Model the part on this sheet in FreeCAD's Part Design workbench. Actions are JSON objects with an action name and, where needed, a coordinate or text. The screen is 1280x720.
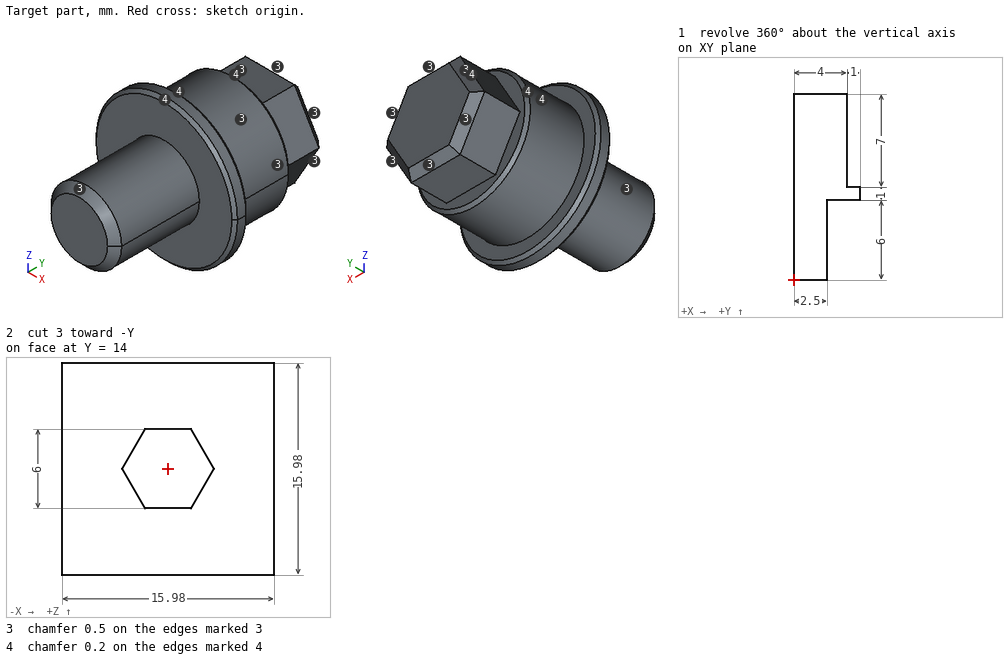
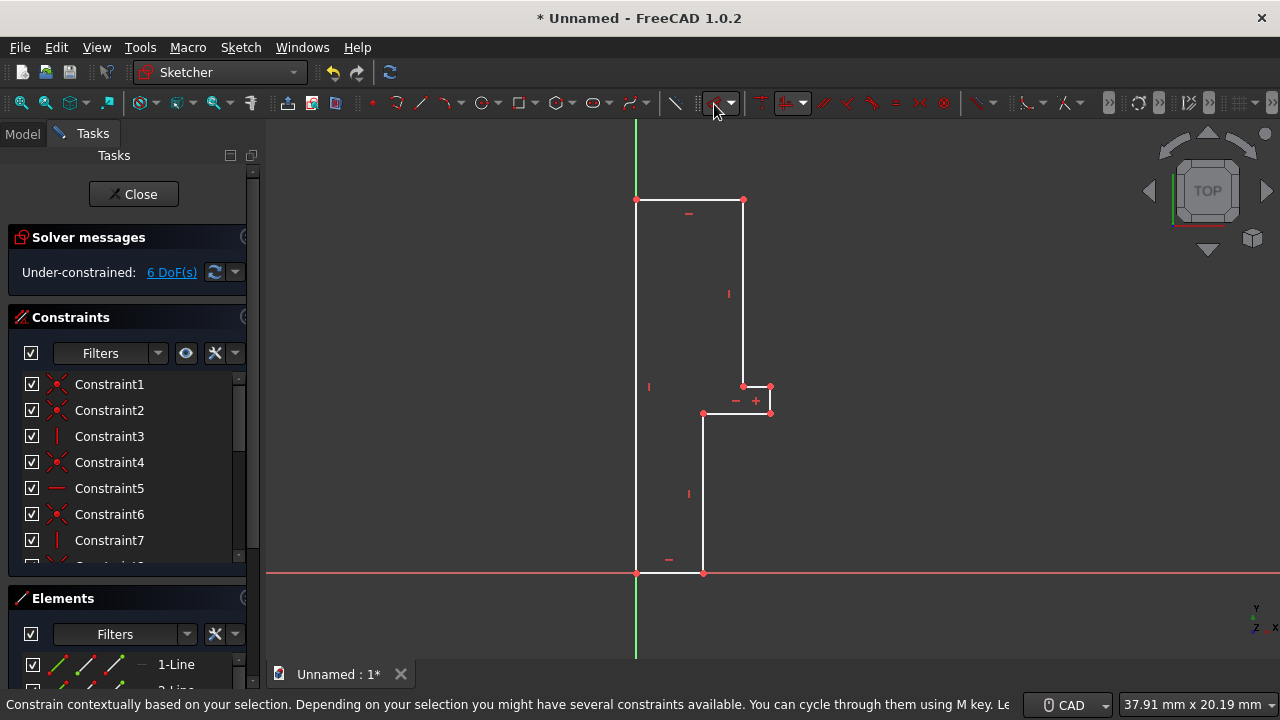
{"action": "left_click", "coordinate": [703, 525]}
{"action": "left_click", "coordinate": [669, 494]}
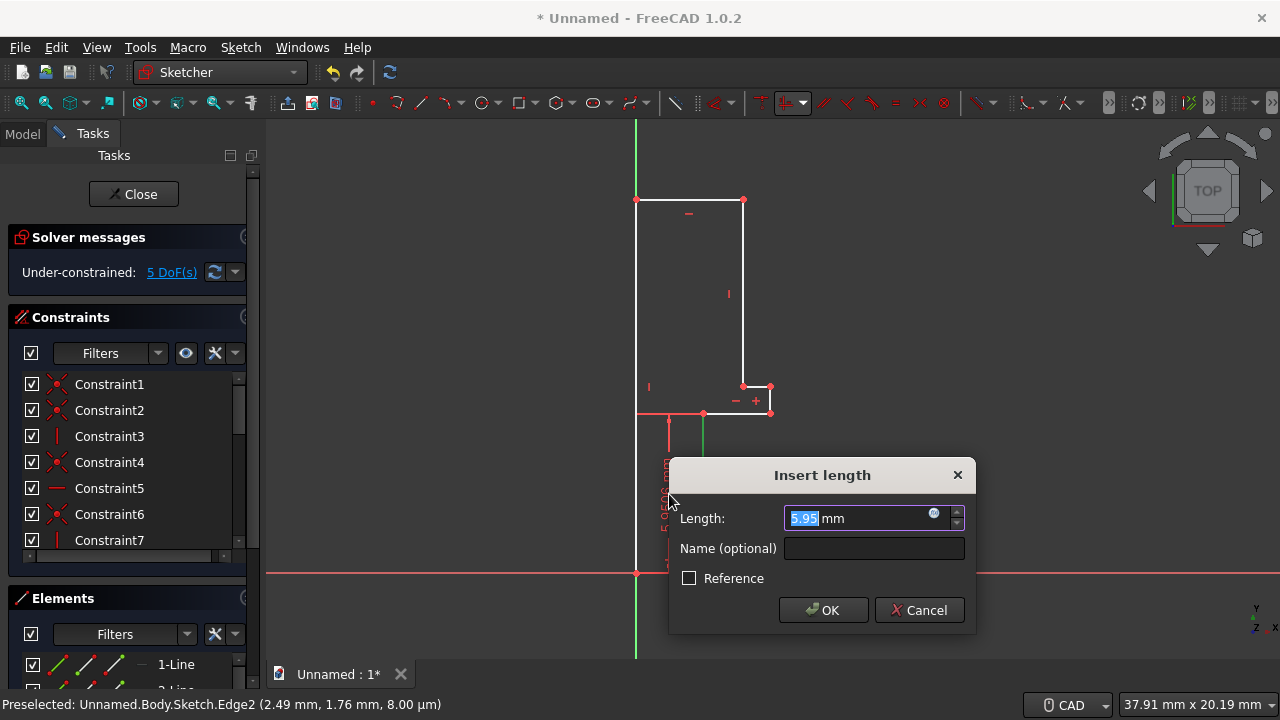
{"action": "type", "text": "6"}
{"action": "key", "text": "Return"}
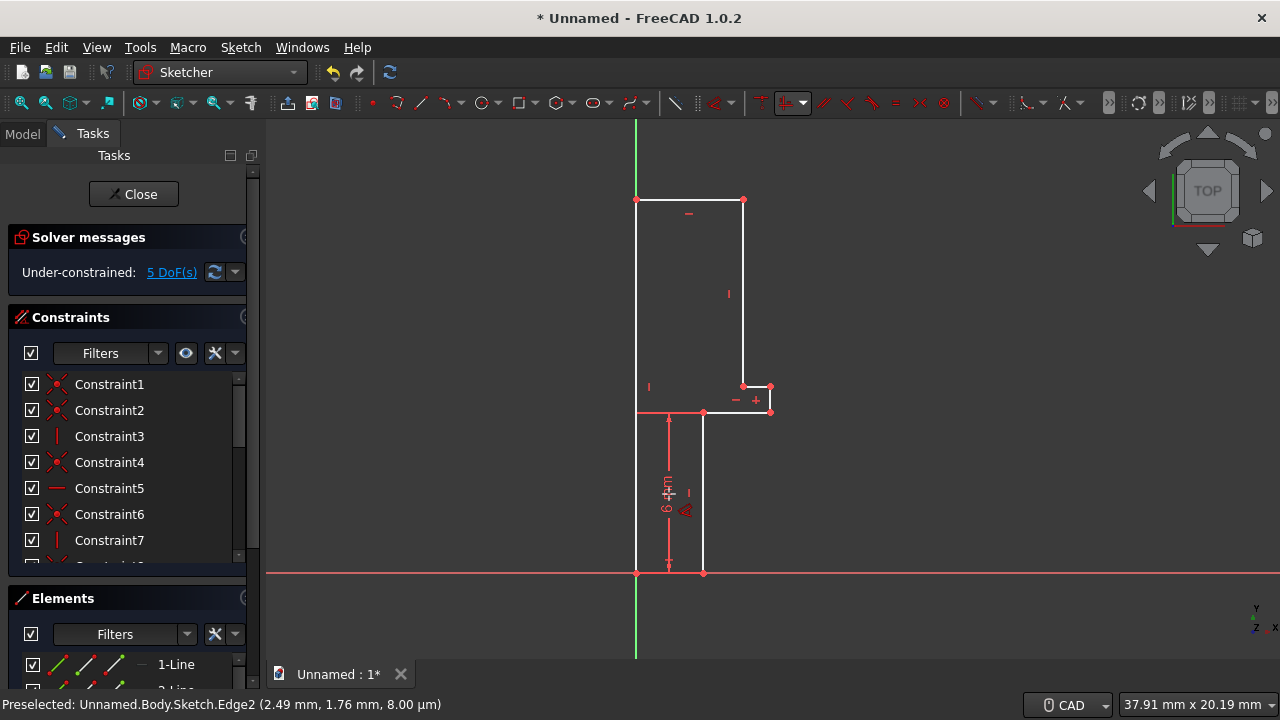
{"action": "scroll", "coordinate": [770, 402], "scroll_direction": "up", "scroll_amount": 2}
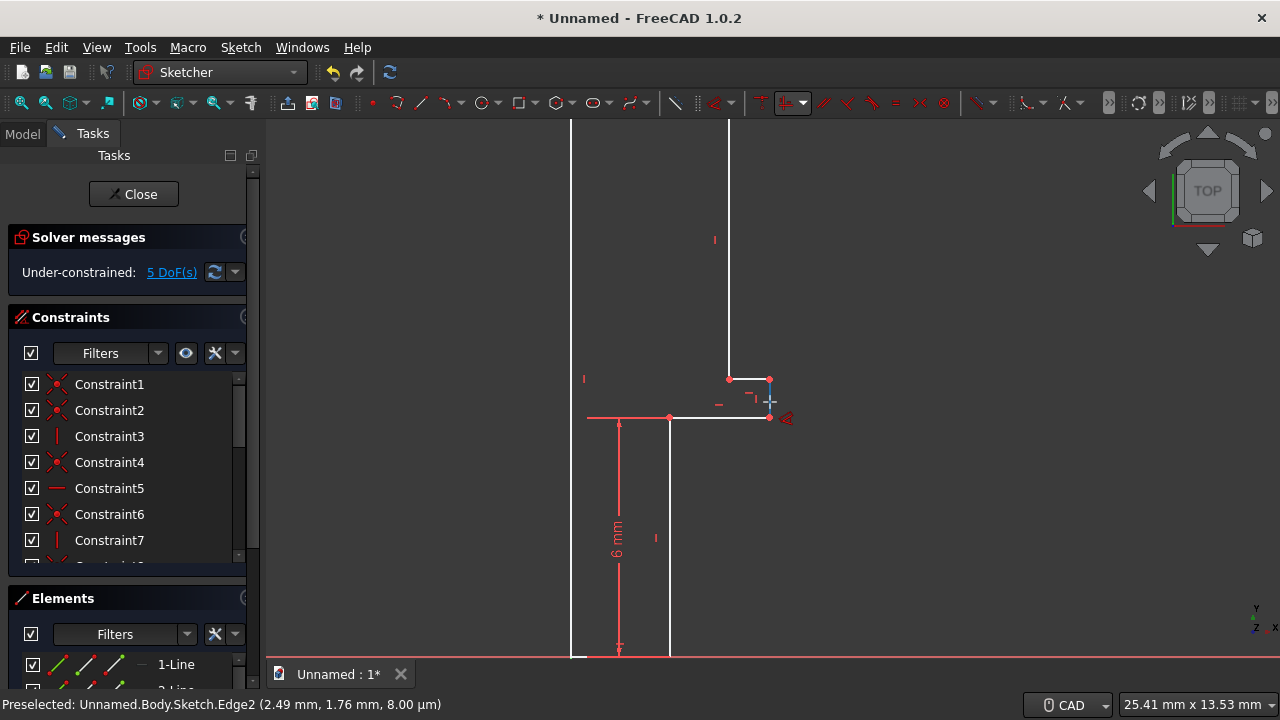
{"action": "left_click", "coordinate": [770, 402]}
{"action": "left_click", "coordinate": [804, 399]}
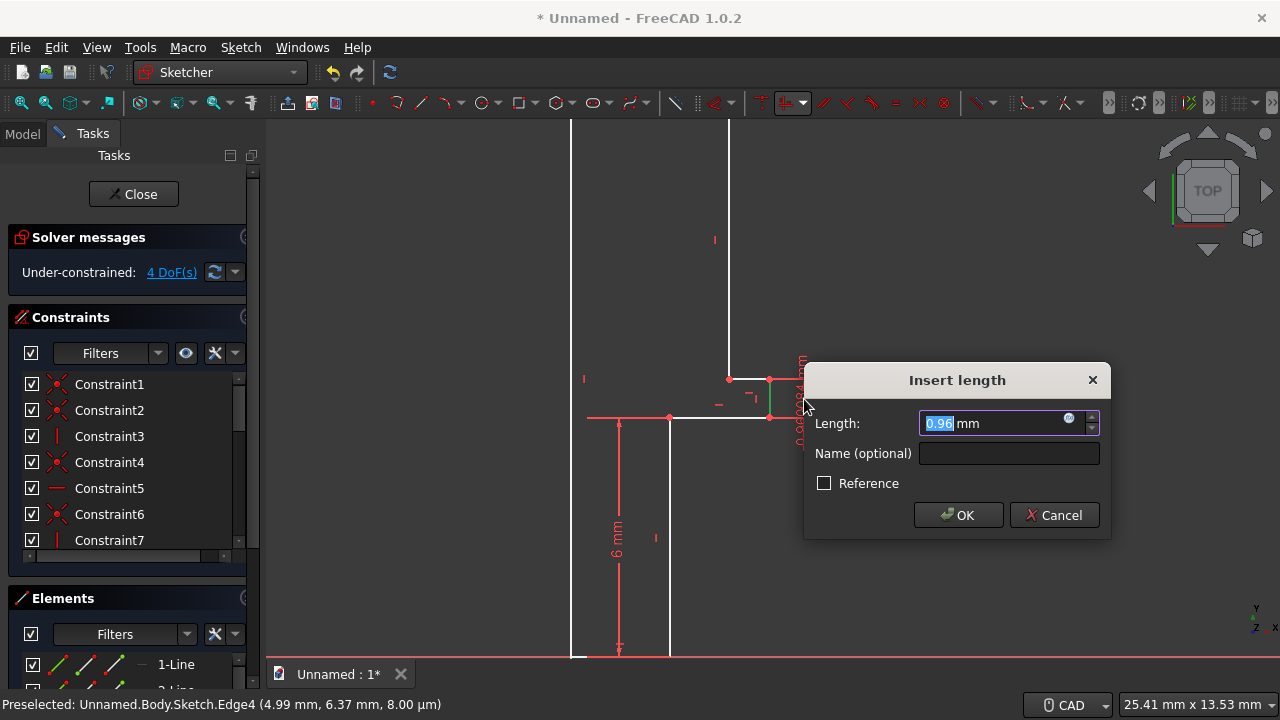
{"action": "type", "text": "1"}
{"action": "key", "text": "Return"}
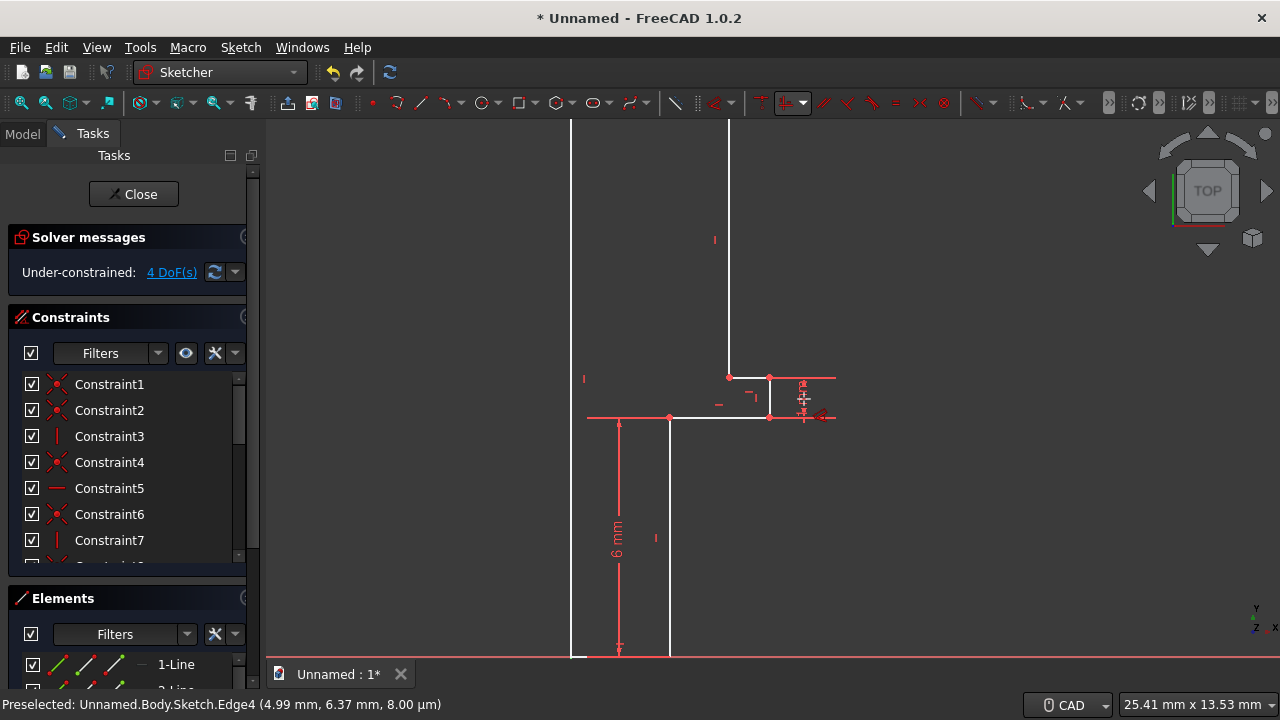
{"action": "left_click", "coordinate": [758, 378]}
{"action": "left_click", "coordinate": [750, 344]}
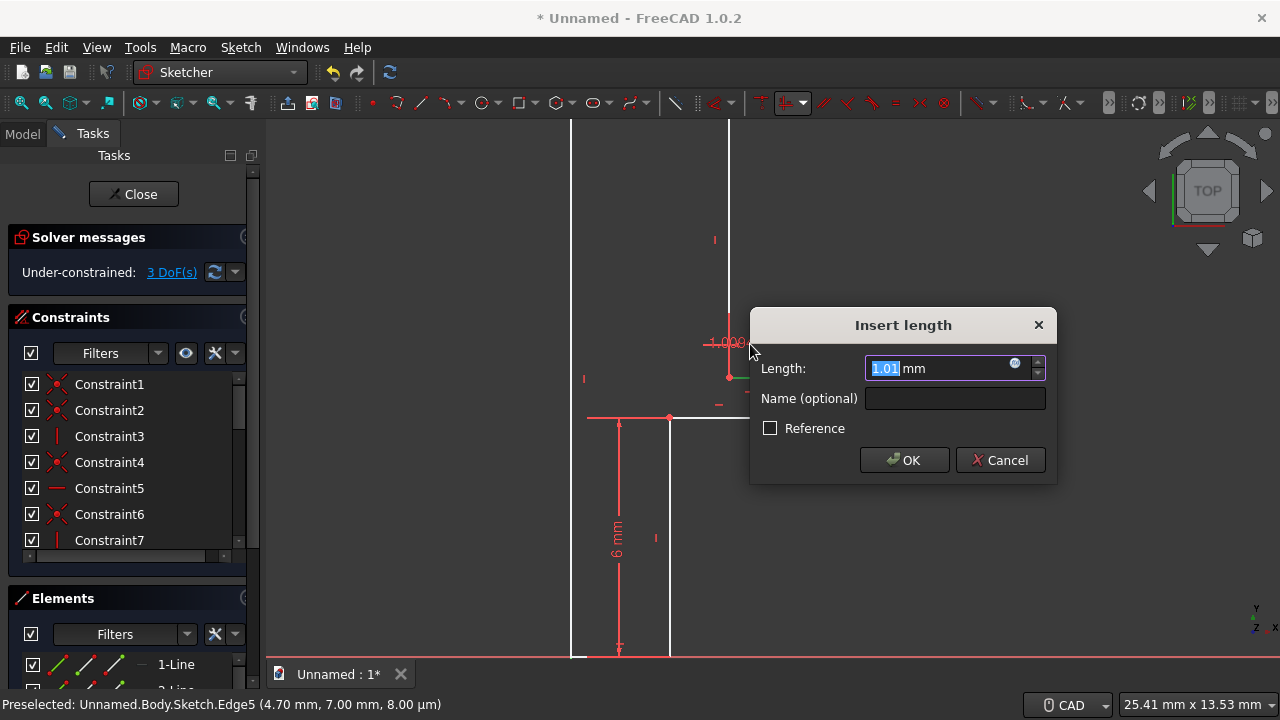
{"action": "type", "text": "1"}
{"action": "key", "text": "Return"}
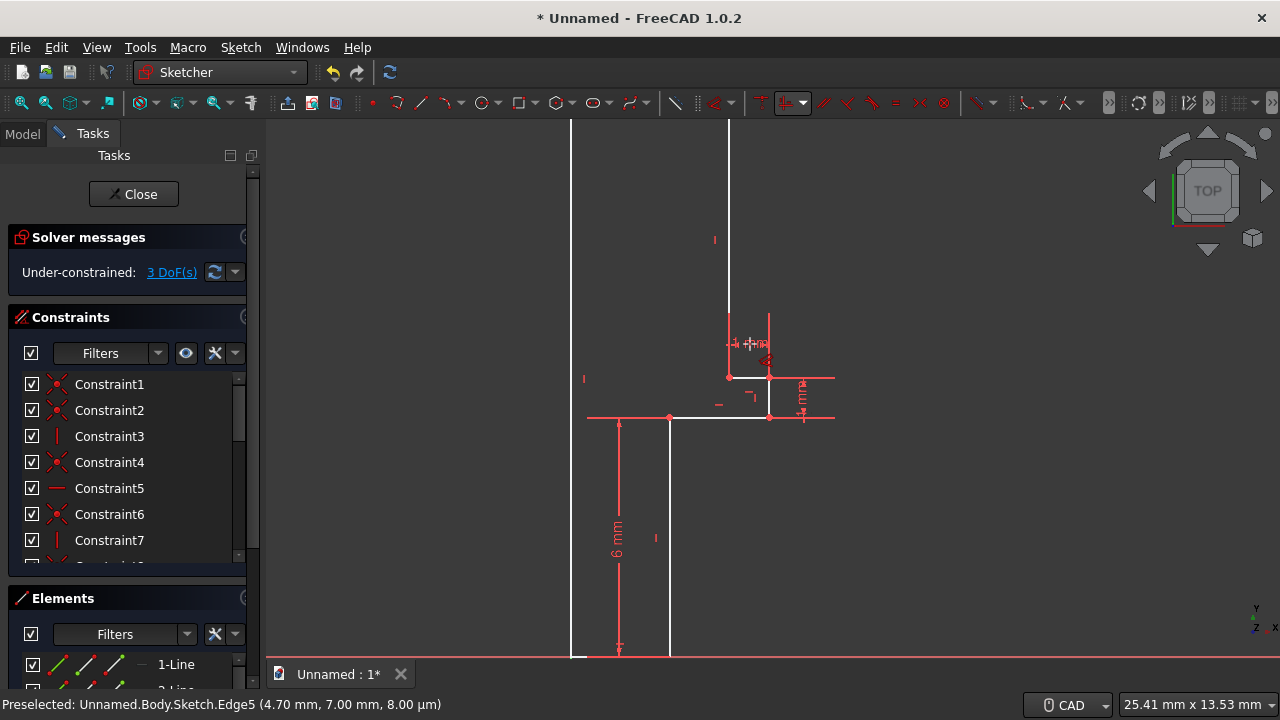
{"action": "left_click", "coordinate": [729, 295]}
{"action": "left_click", "coordinate": [763, 262]}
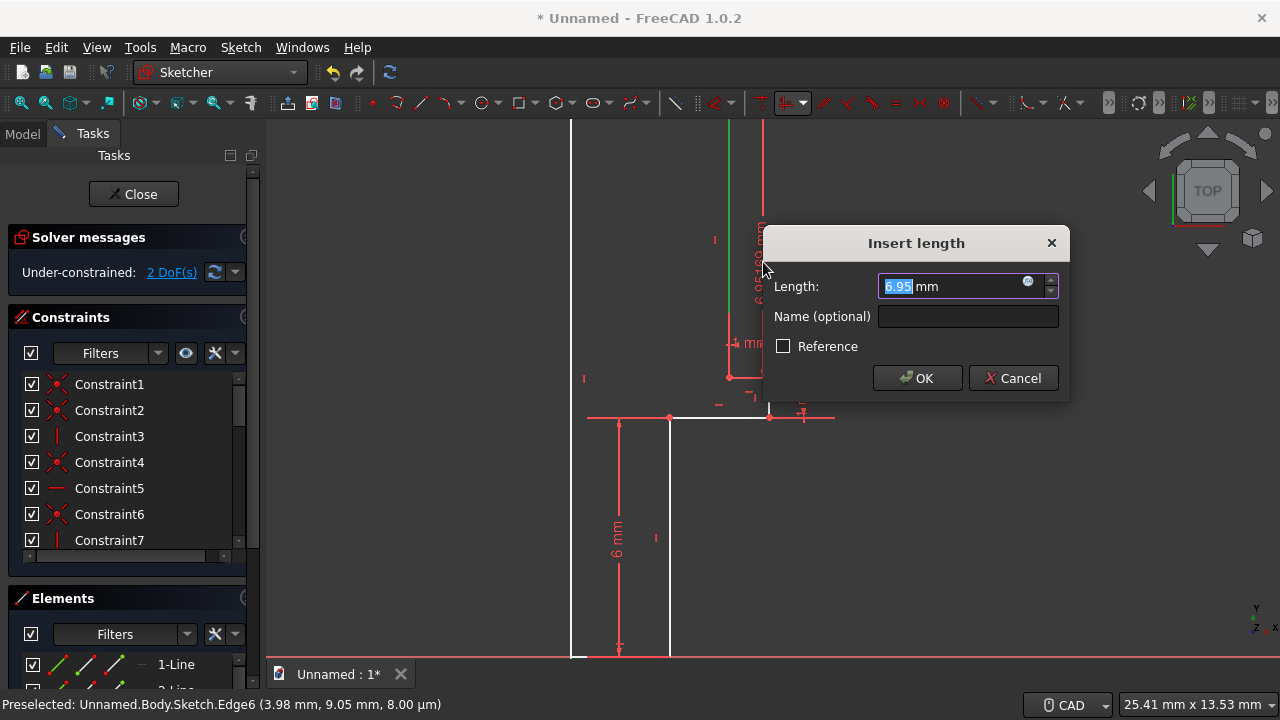
{"action": "type", "text": "7"}
{"action": "key", "text": "Return"}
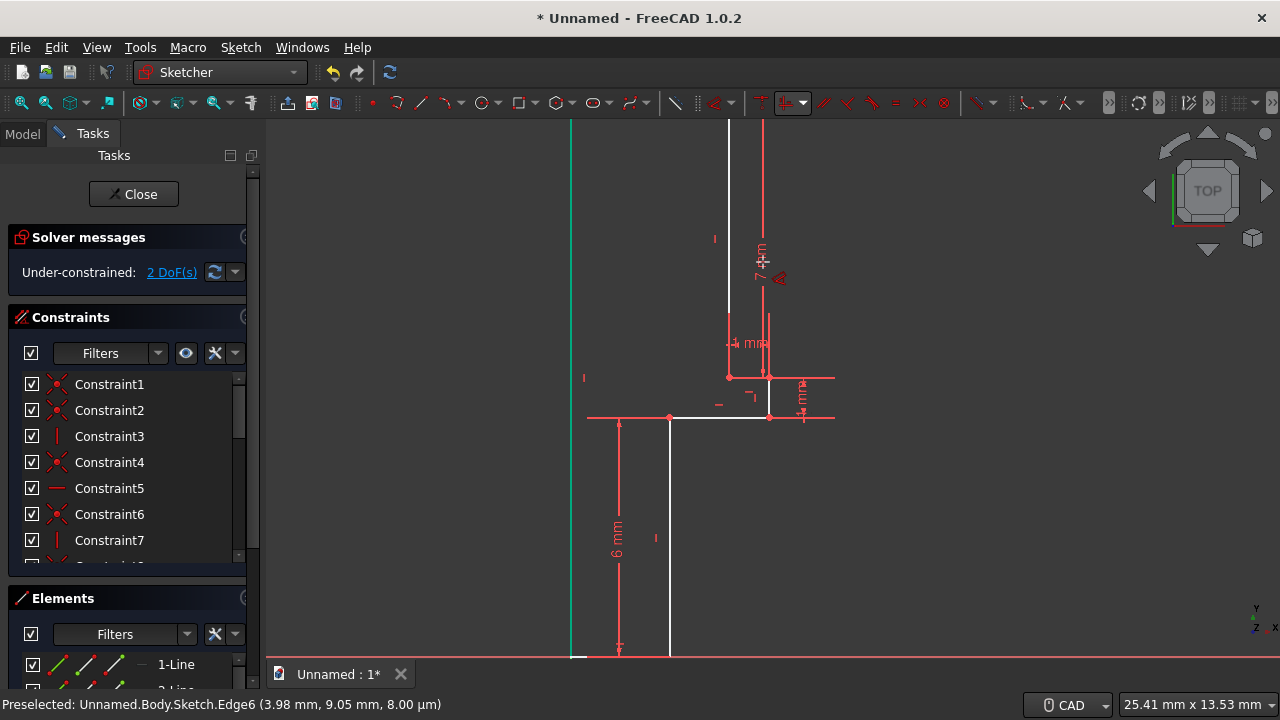
{"action": "scroll", "coordinate": [774, 412], "scroll_direction": "down", "scroll_amount": 2}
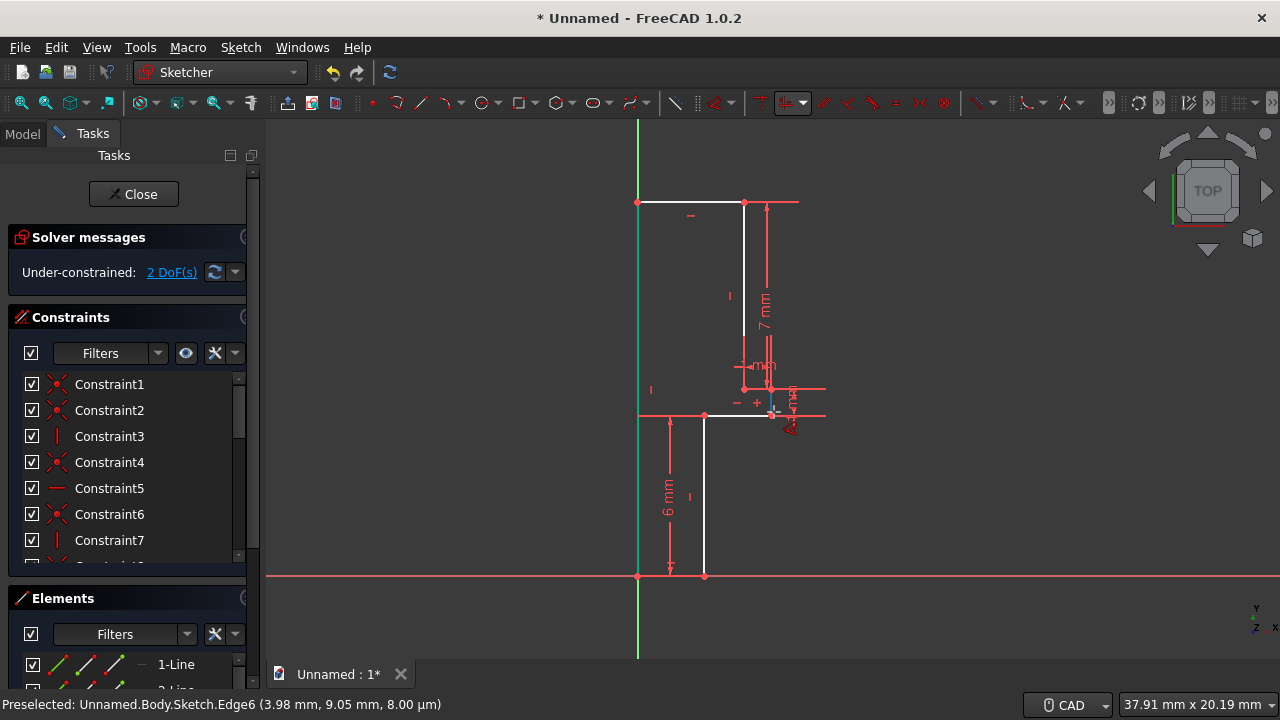
{"action": "left_click", "coordinate": [712, 202]}
{"action": "left_click", "coordinate": [691, 168]}